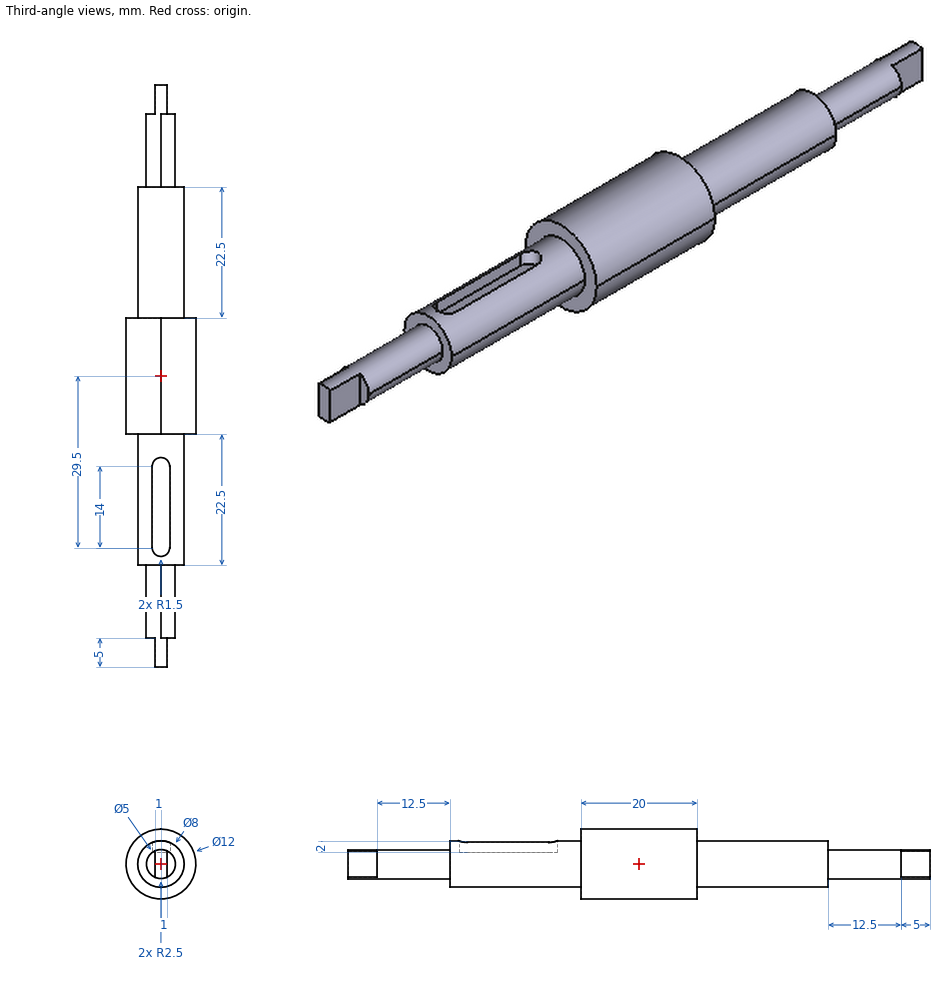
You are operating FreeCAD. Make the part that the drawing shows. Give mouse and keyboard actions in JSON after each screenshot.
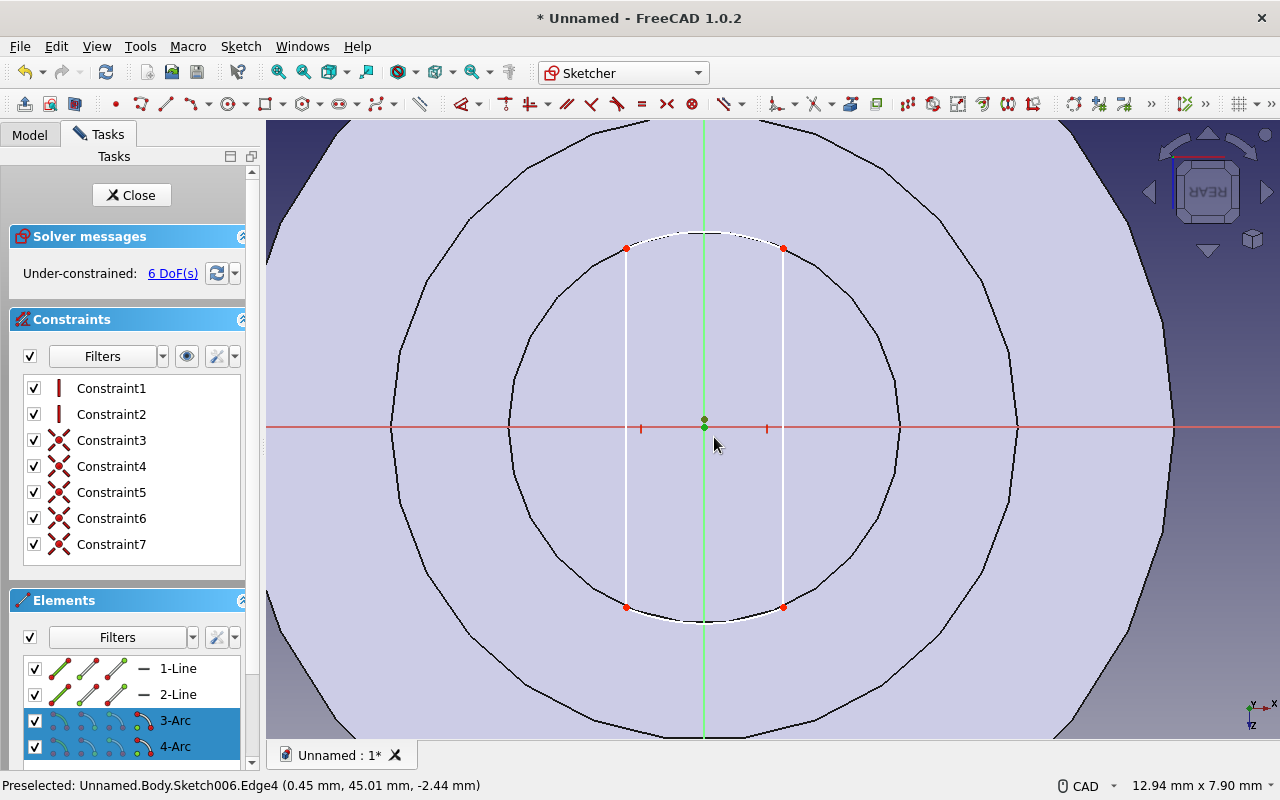
{"action": "key", "text": "c"}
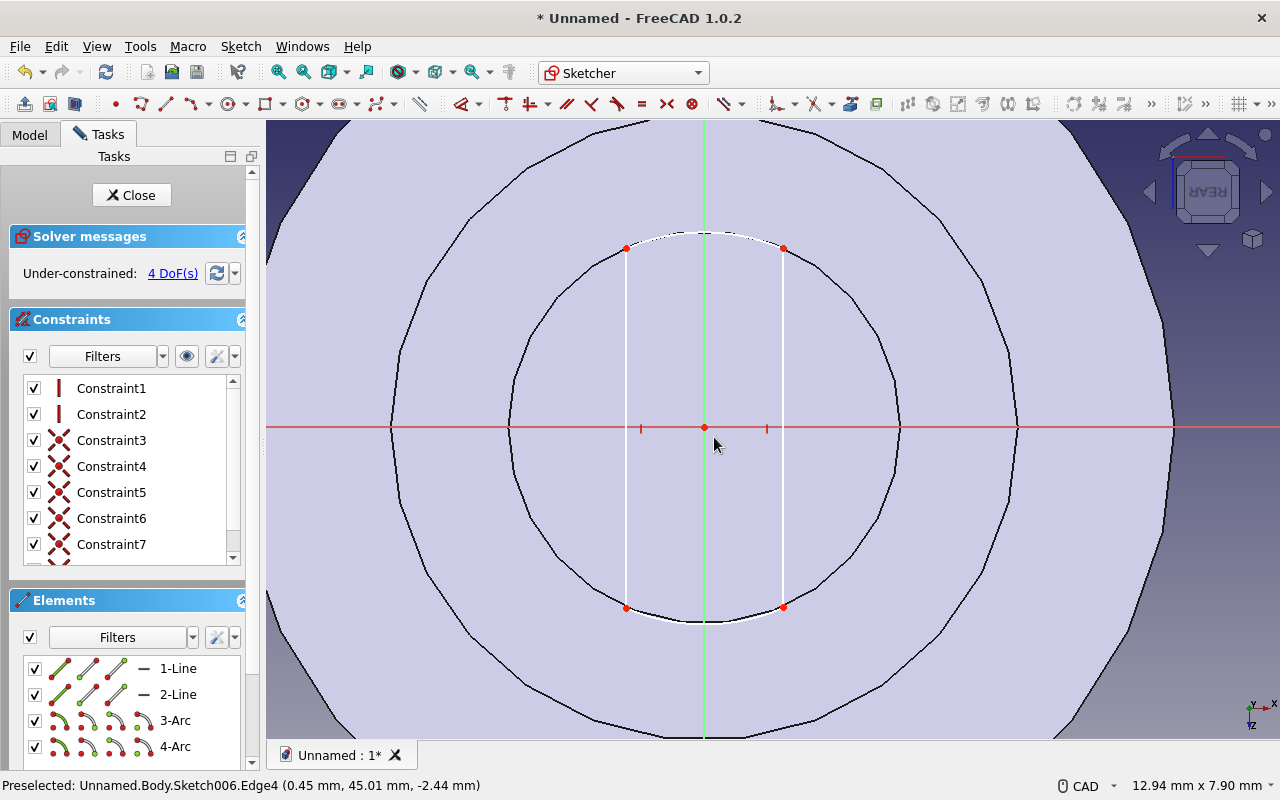
{"action": "left_click", "coordinate": [672, 622]}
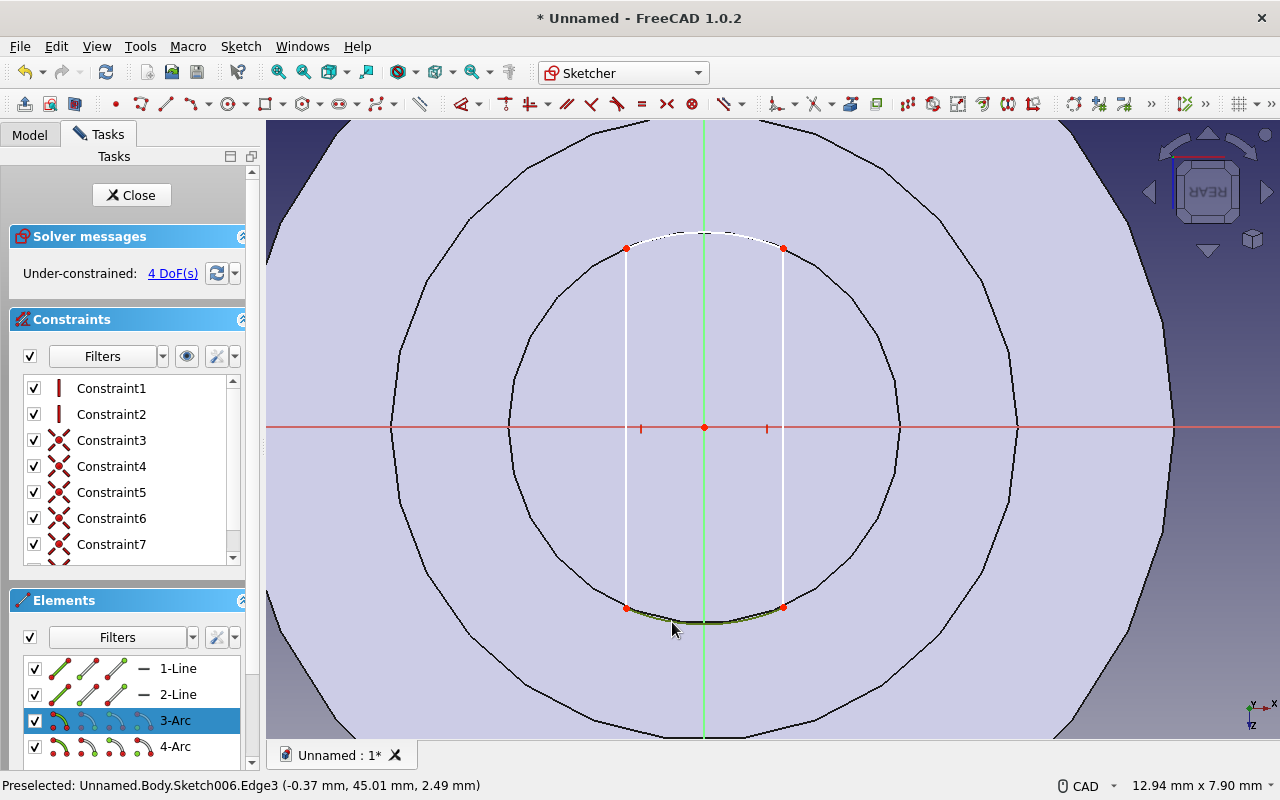
{"action": "left_click", "coordinate": [737, 235]}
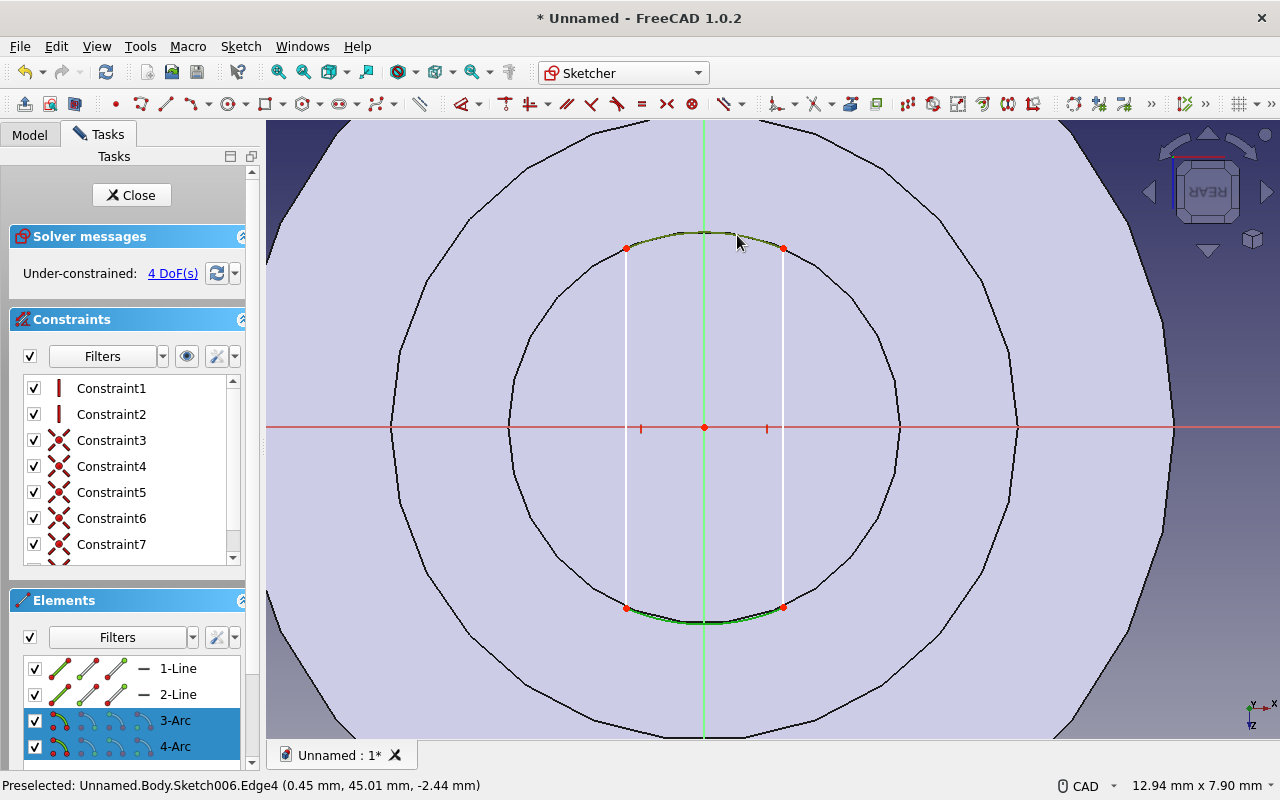
{"action": "key", "text": "e"}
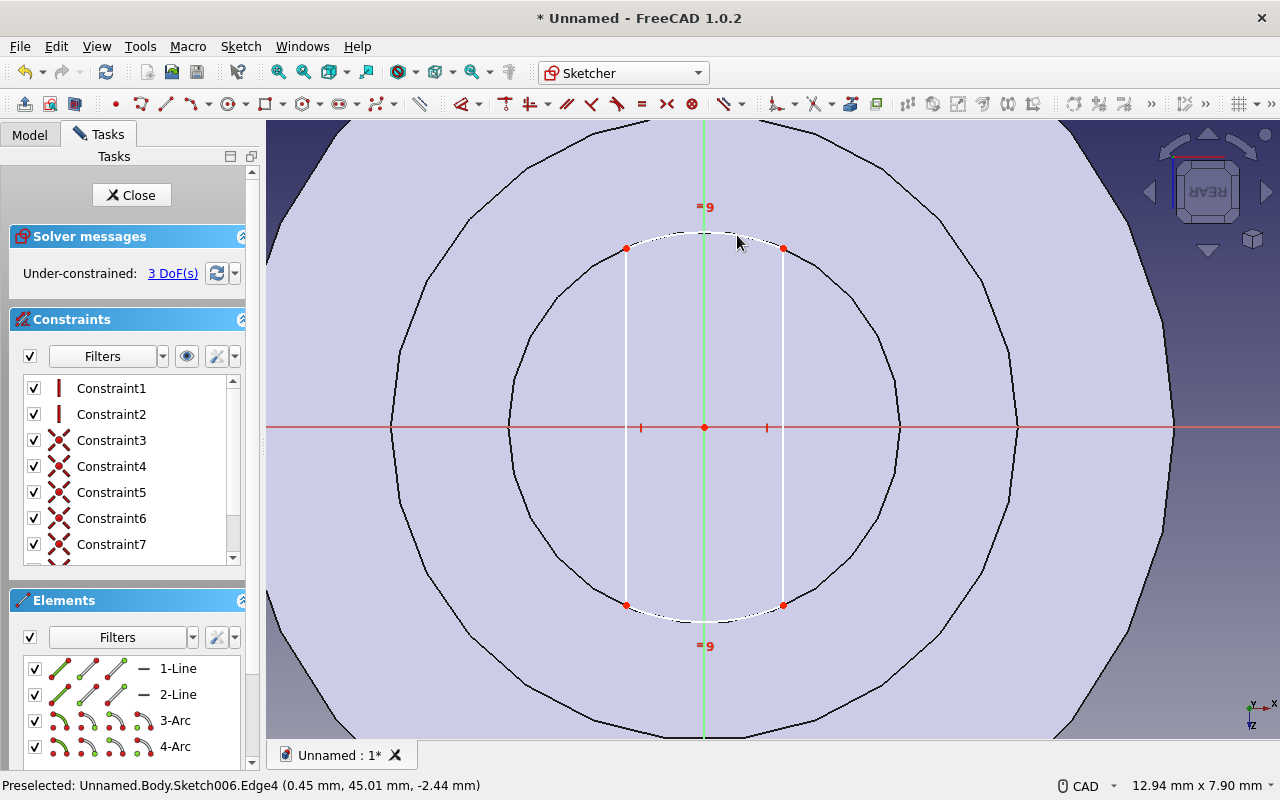
{"action": "key", "text": "d"}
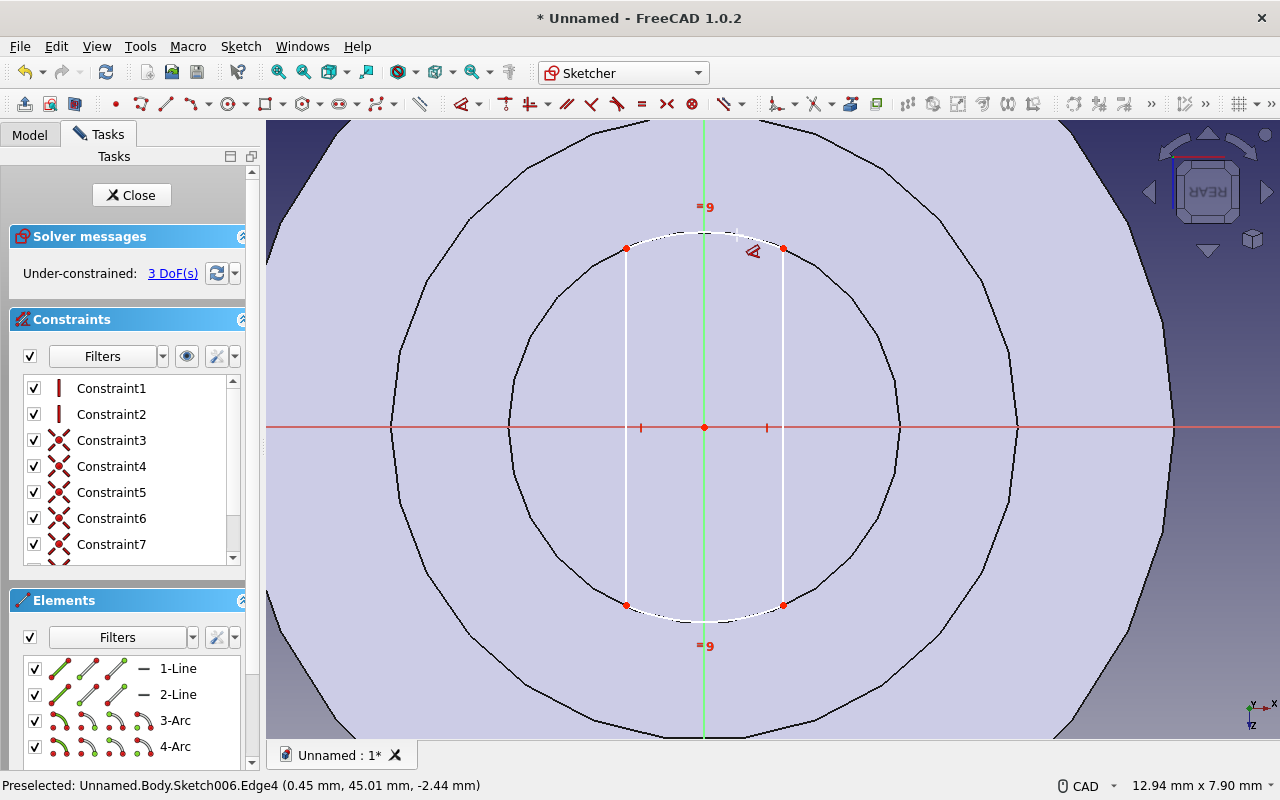
{"action": "left_click", "coordinate": [672, 619]}
{"action": "left_click", "coordinate": [667, 651]}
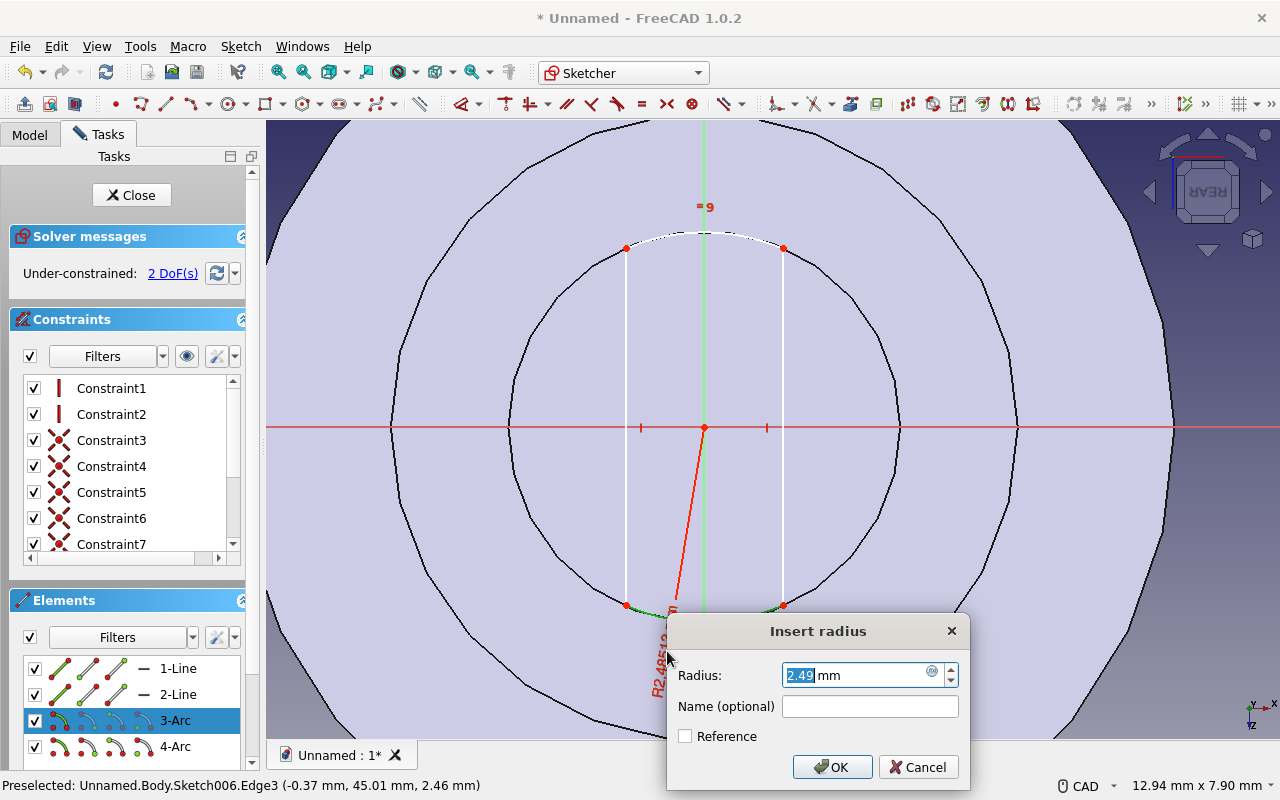
{"action": "type", "text": "2.5"}
{"action": "key", "text": "Return"}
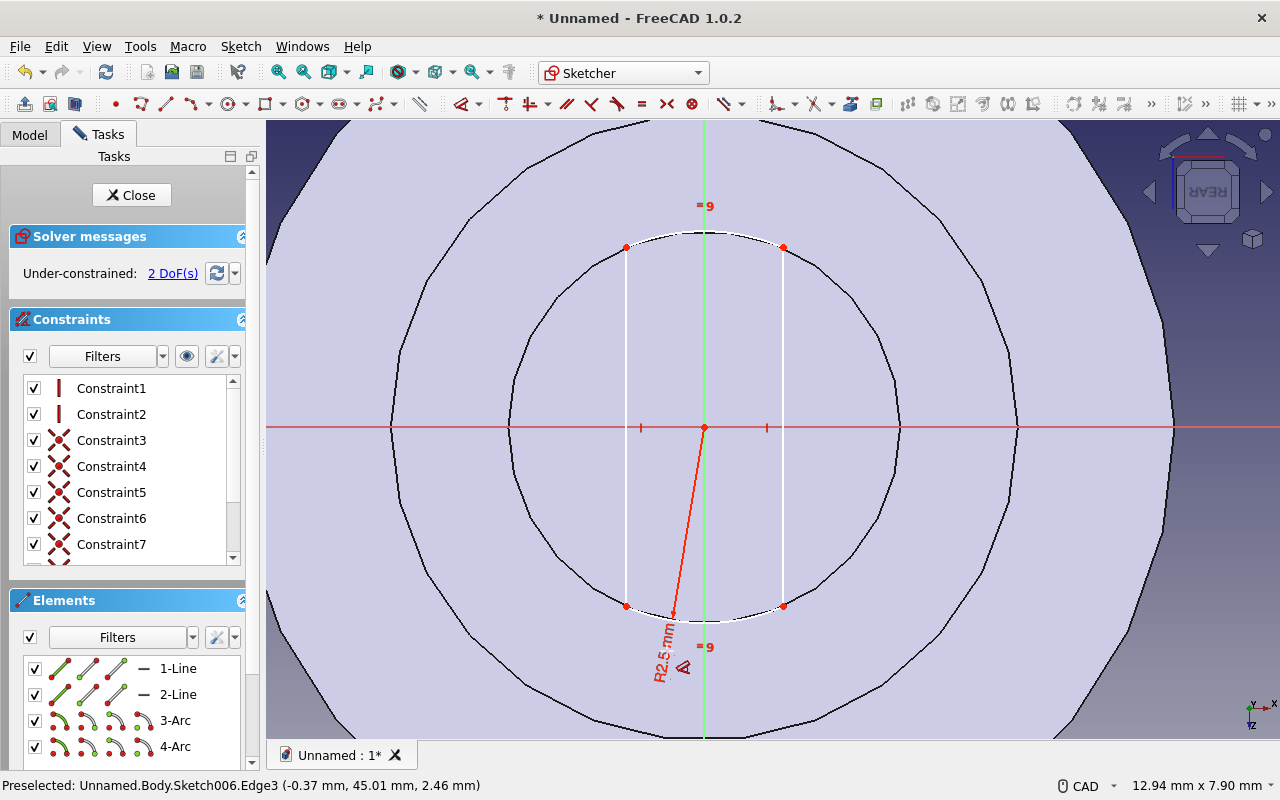
{"action": "left_click", "coordinate": [626, 248]}
{"action": "left_click", "coordinate": [665, 214]}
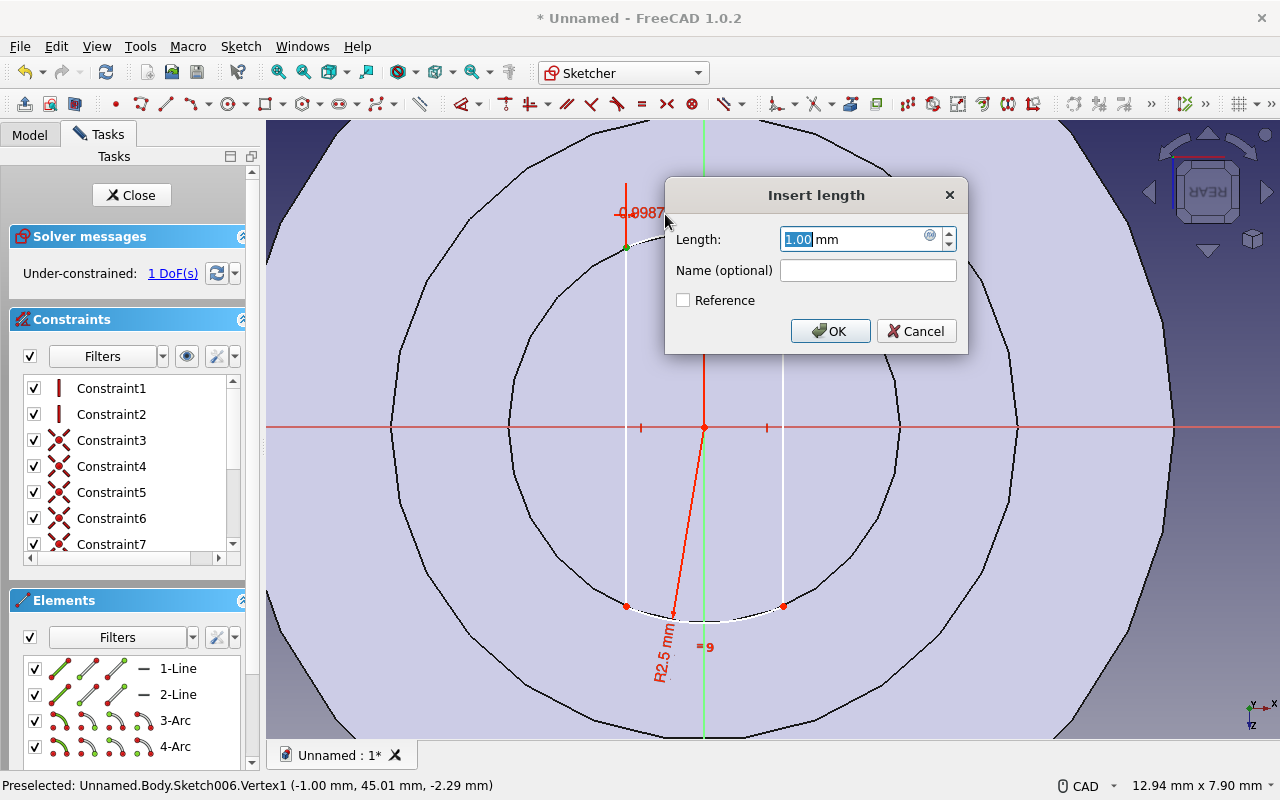
{"action": "type", "text": "1"}
{"action": "key", "text": "Return"}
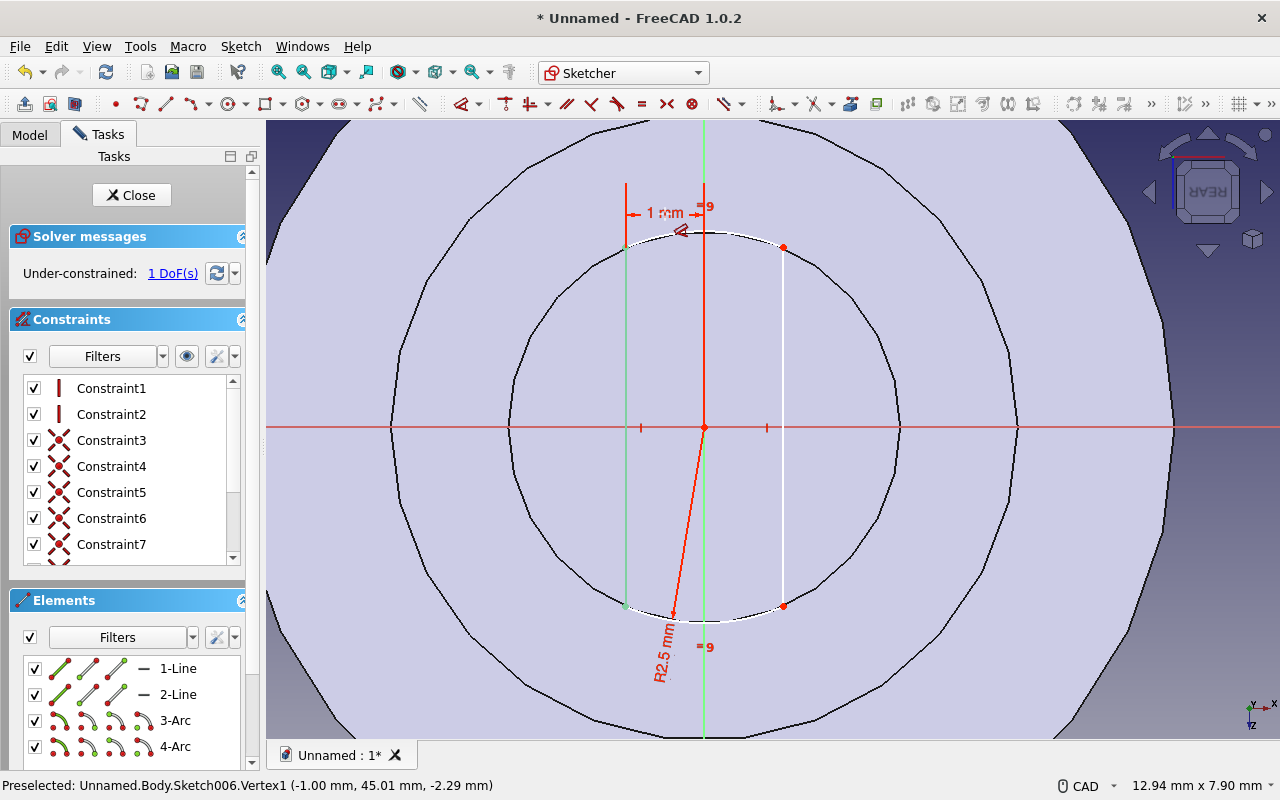
{"action": "left_click", "coordinate": [783, 607]}
{"action": "left_click", "coordinate": [744, 641]}